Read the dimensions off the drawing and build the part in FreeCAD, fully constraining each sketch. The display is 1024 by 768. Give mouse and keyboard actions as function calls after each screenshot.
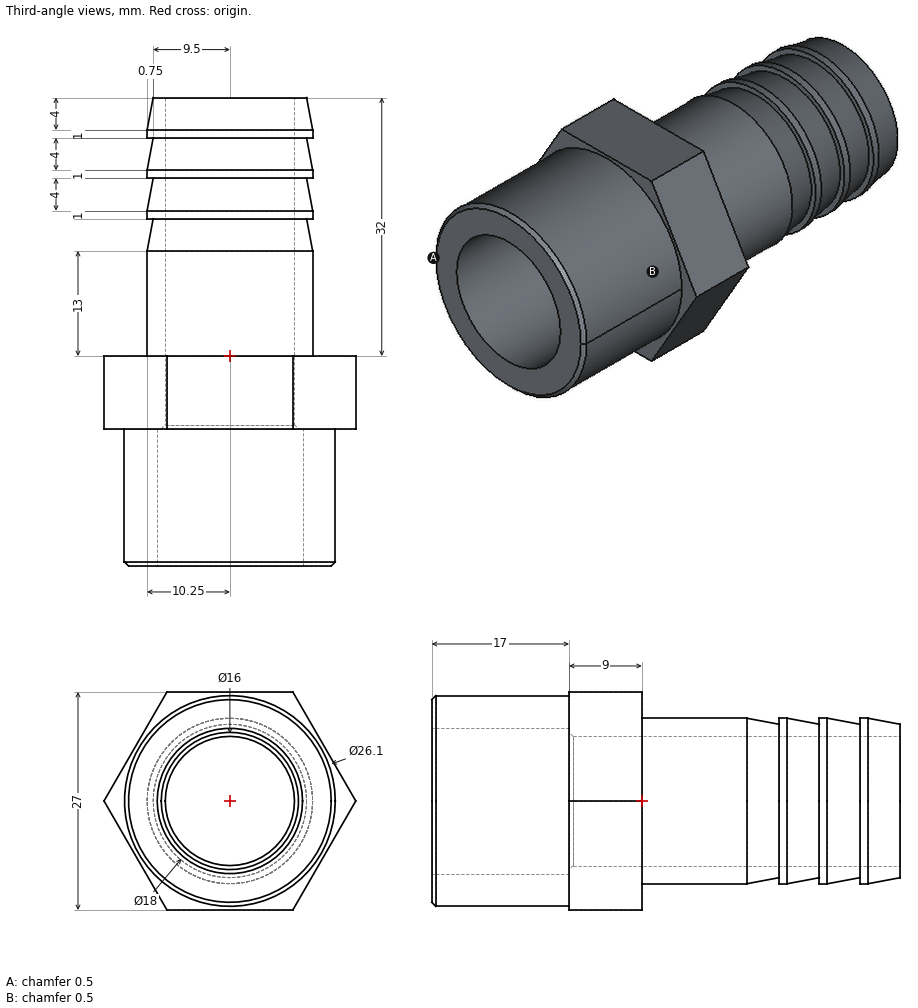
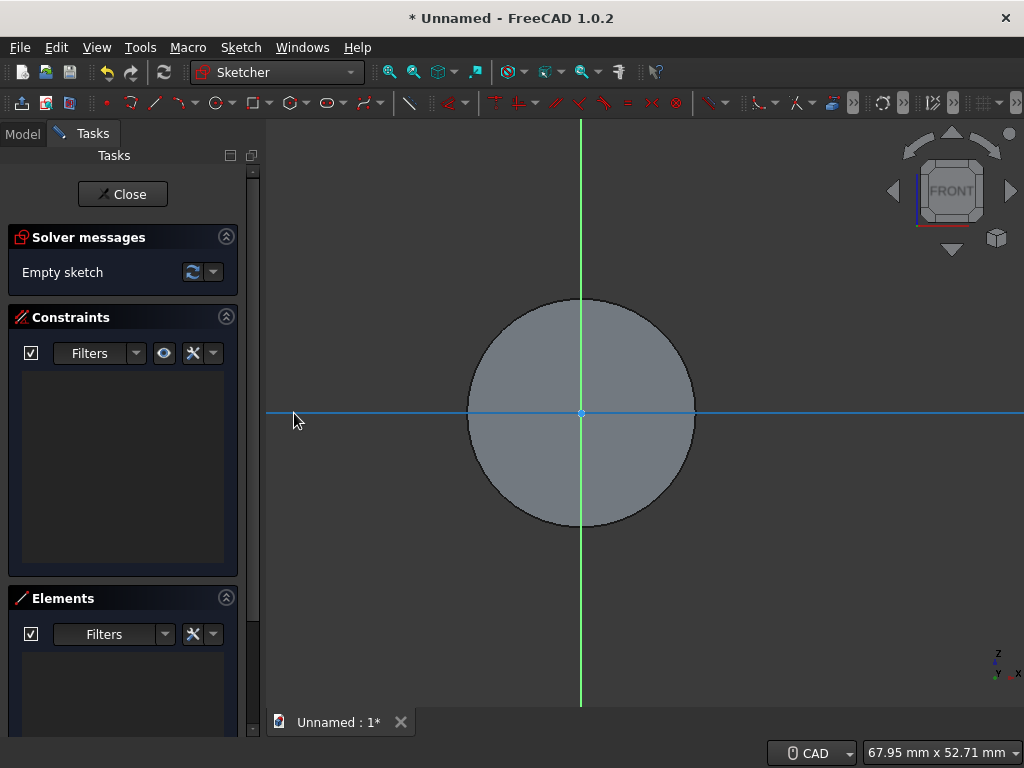
click(290, 104)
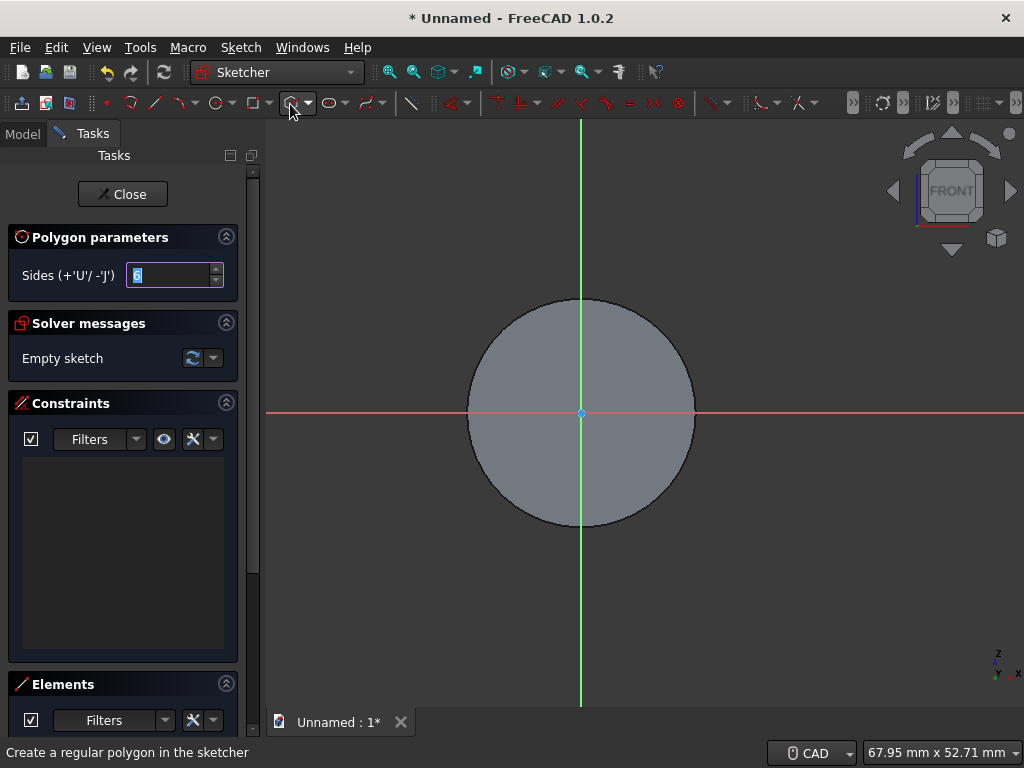
click(581, 413)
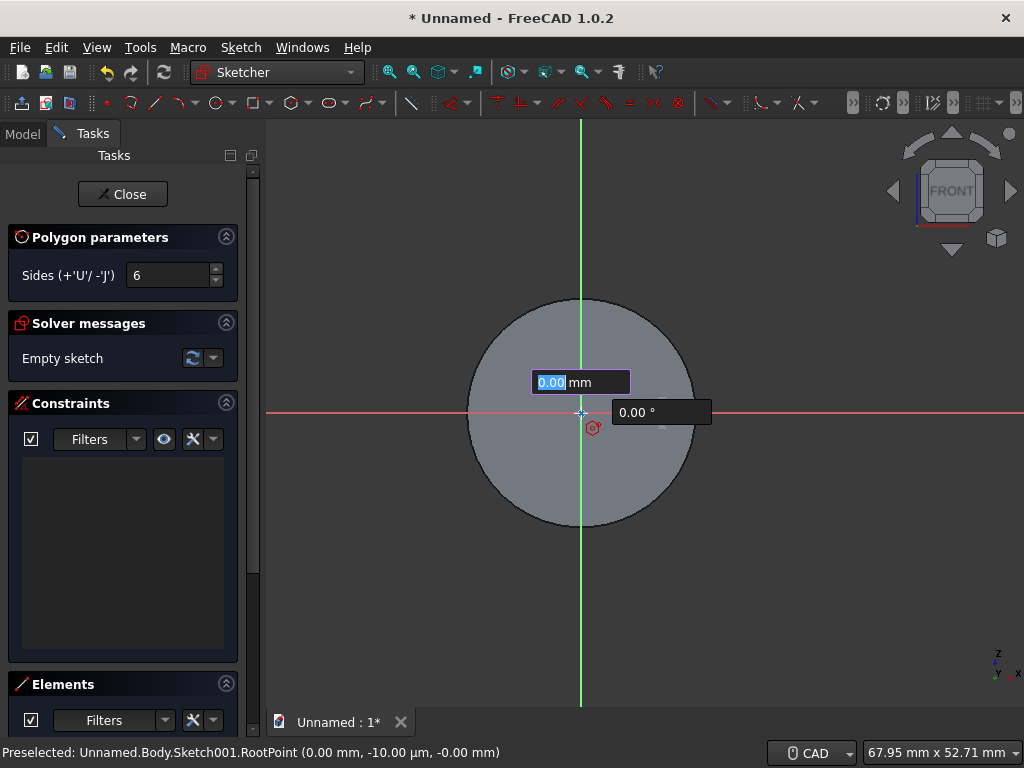
click(755, 413)
right_click(755, 413)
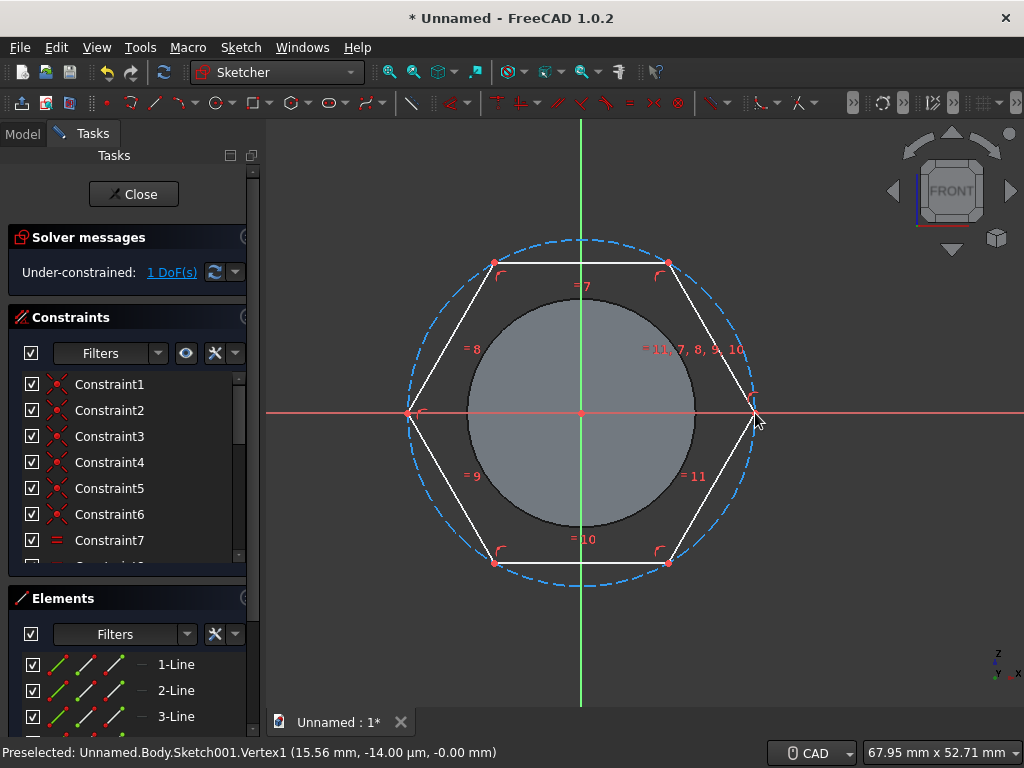
key(d)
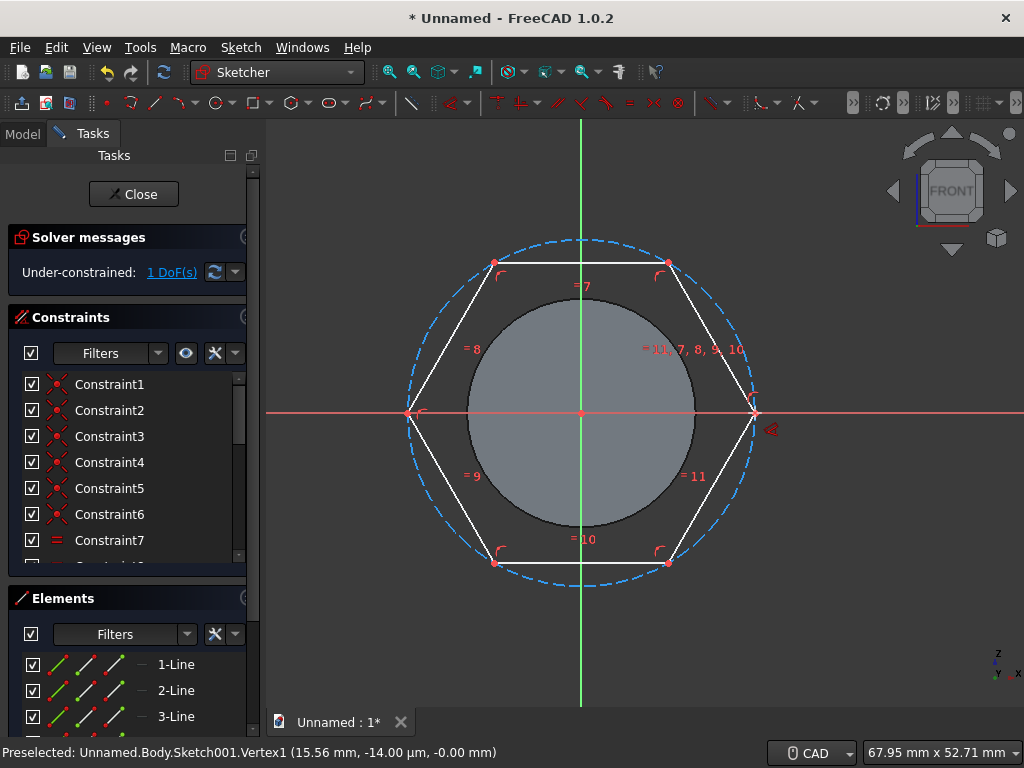
click(495, 563)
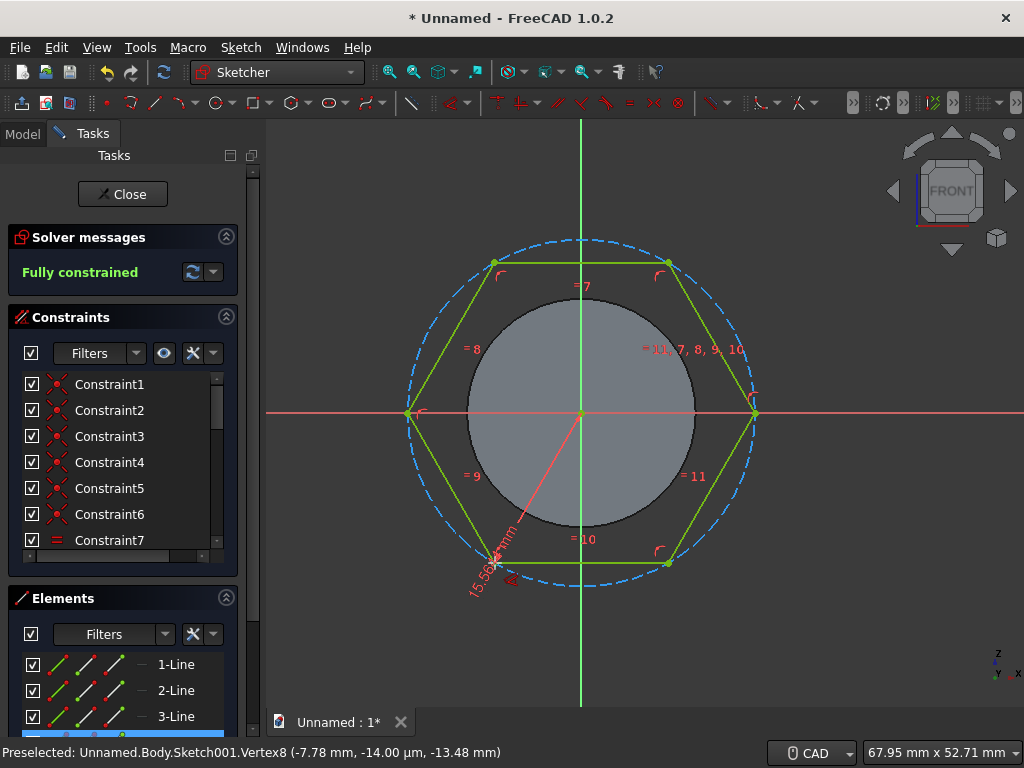
click(668, 263)
click(750, 308)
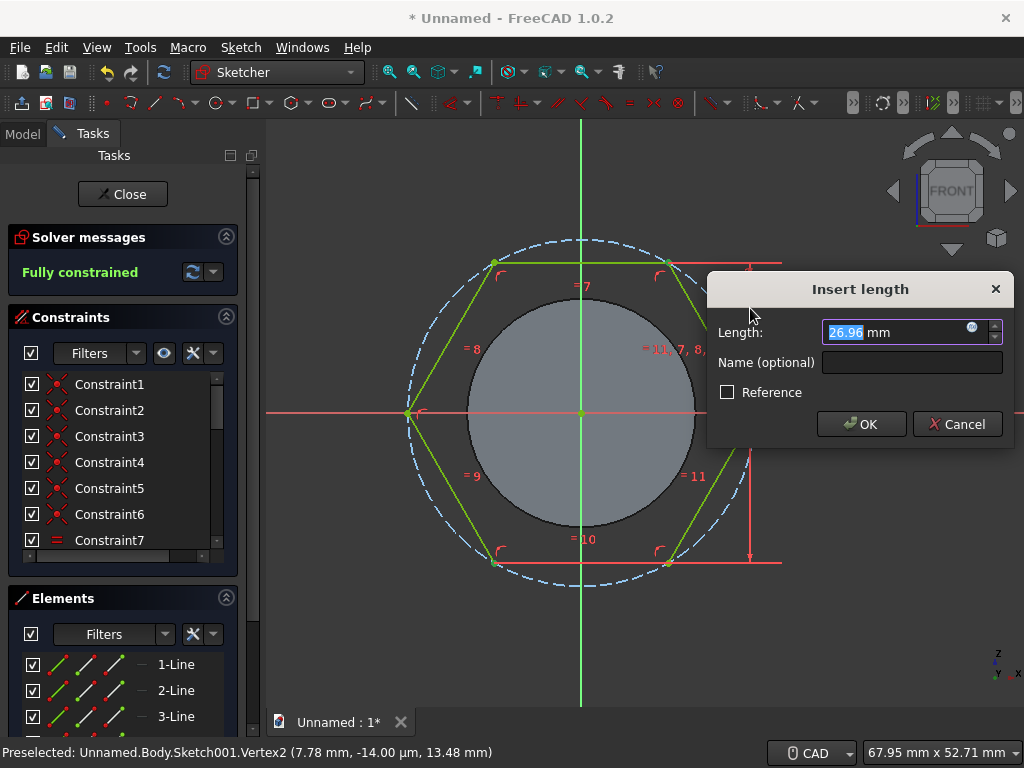
text(27)
key(Return)
key(Escape)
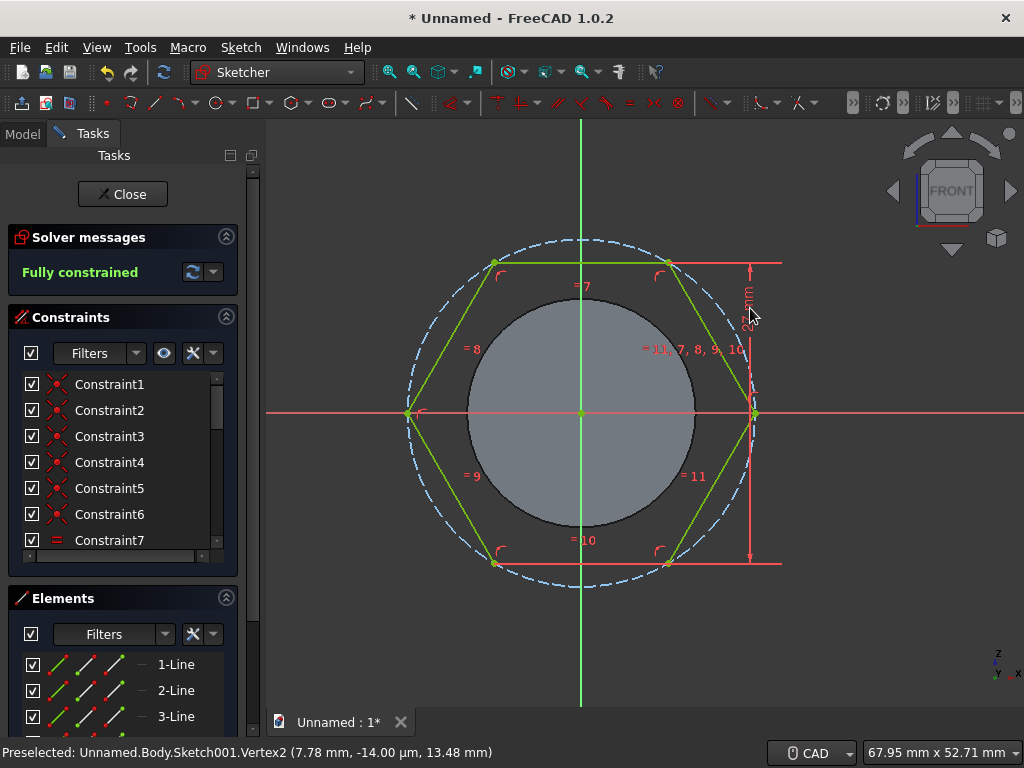
click(123, 194)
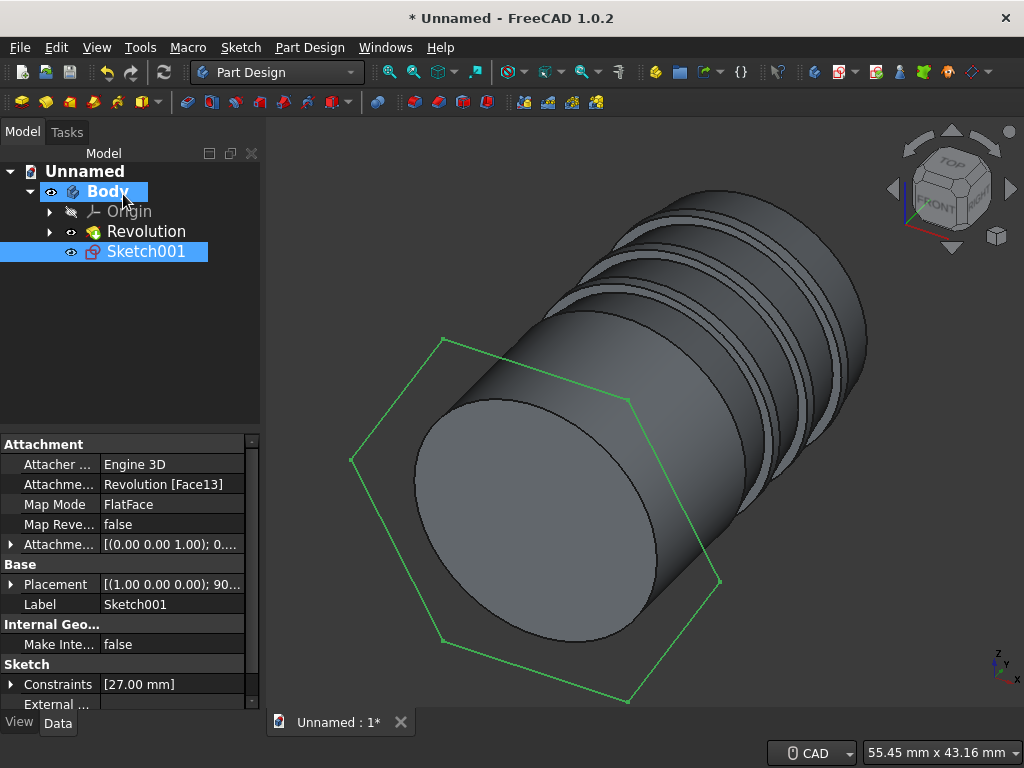
click(22, 102)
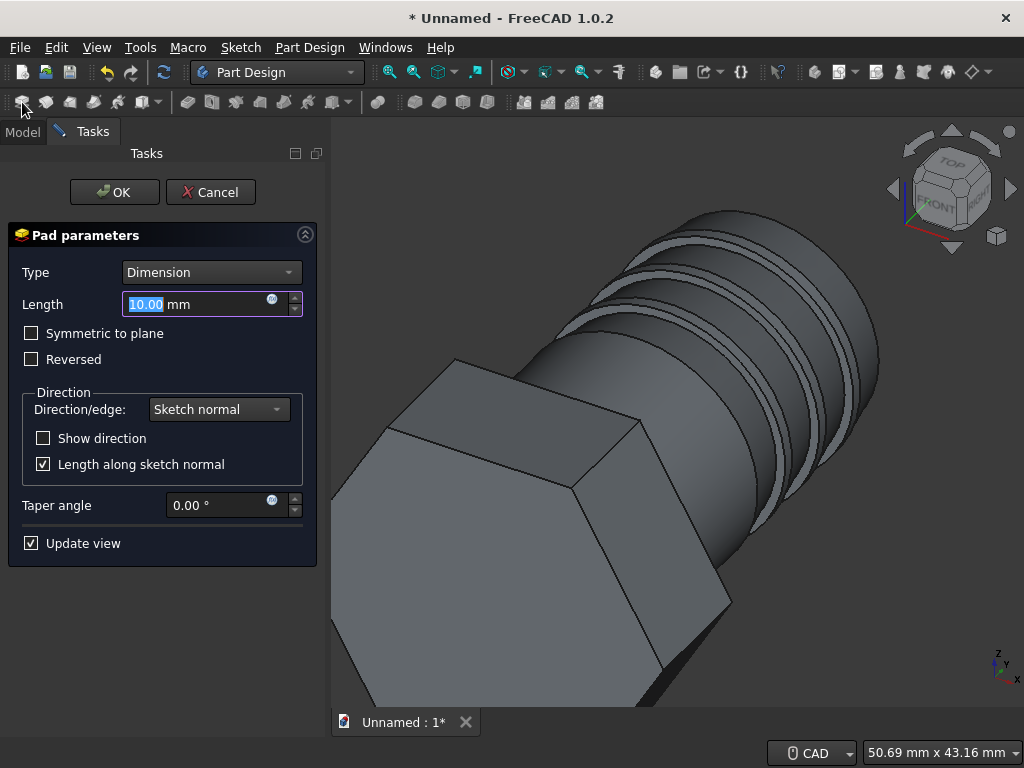
text(9)
key(Tab)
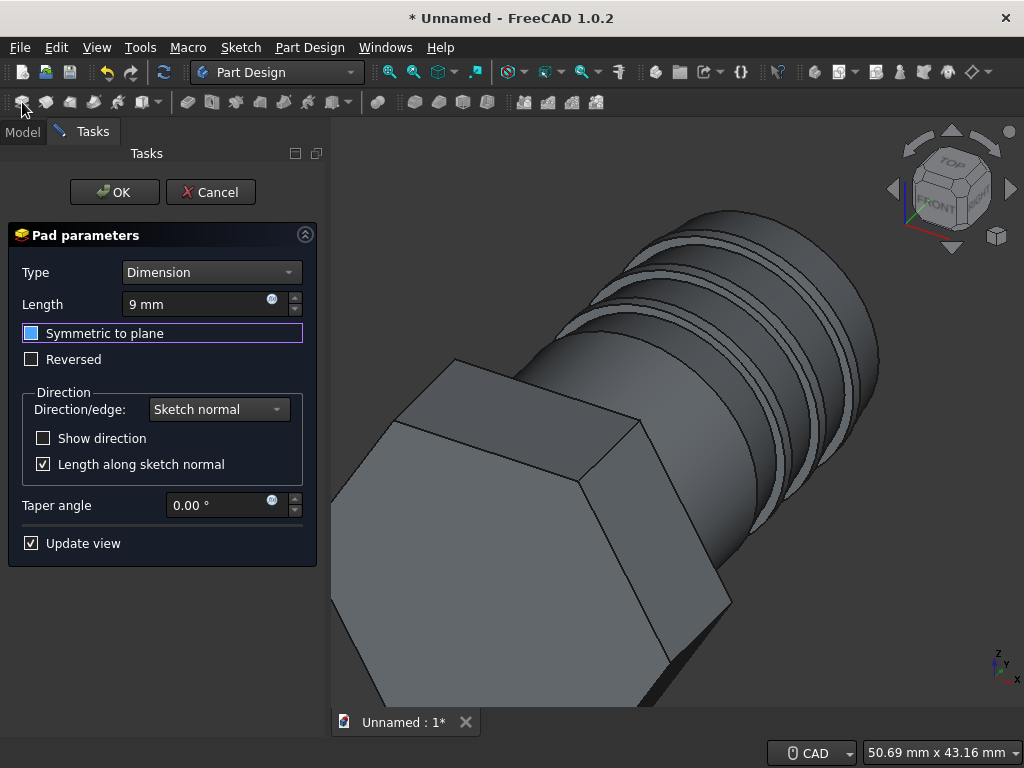
click(115, 192)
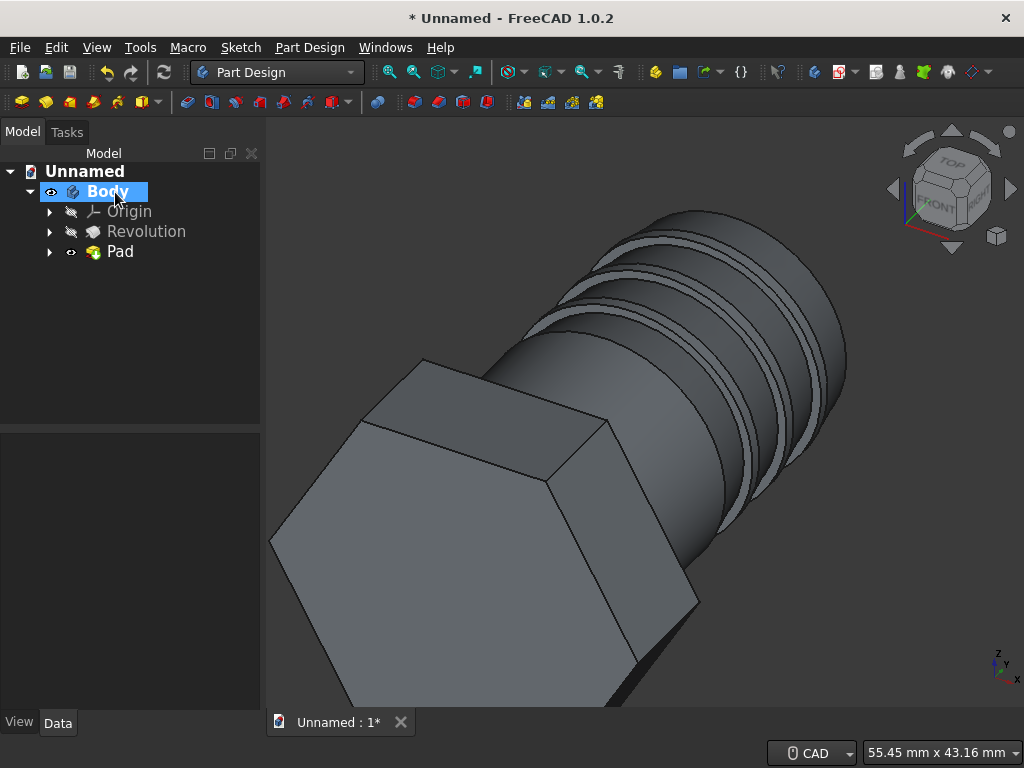
click(390, 72)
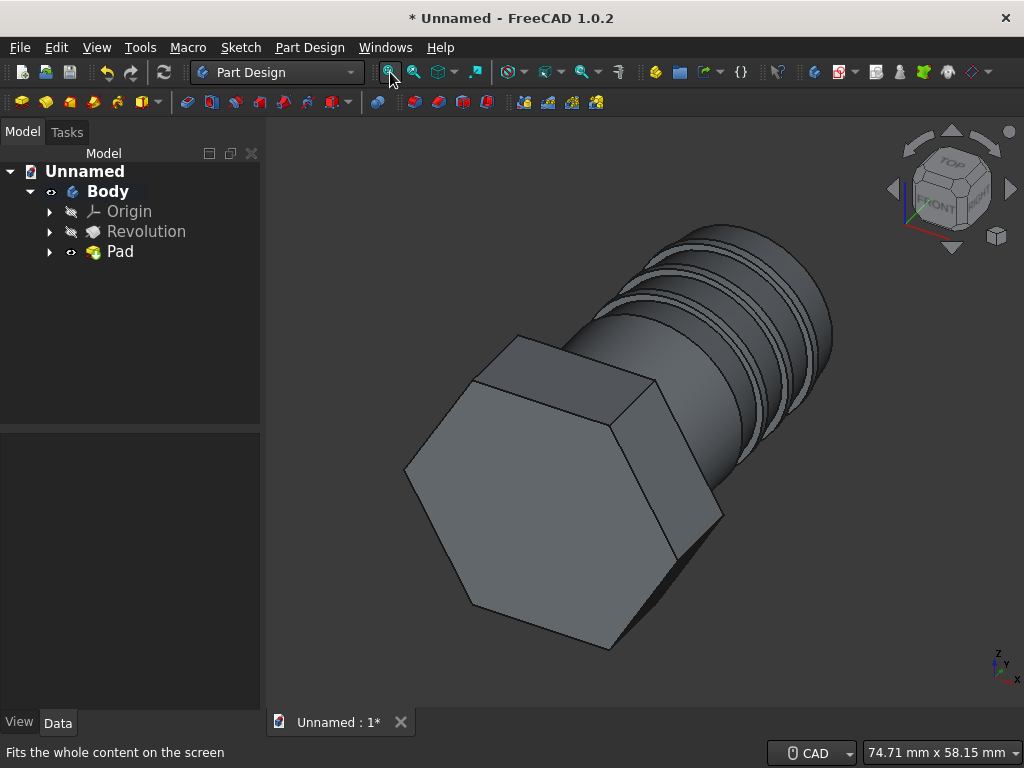
click(541, 514)